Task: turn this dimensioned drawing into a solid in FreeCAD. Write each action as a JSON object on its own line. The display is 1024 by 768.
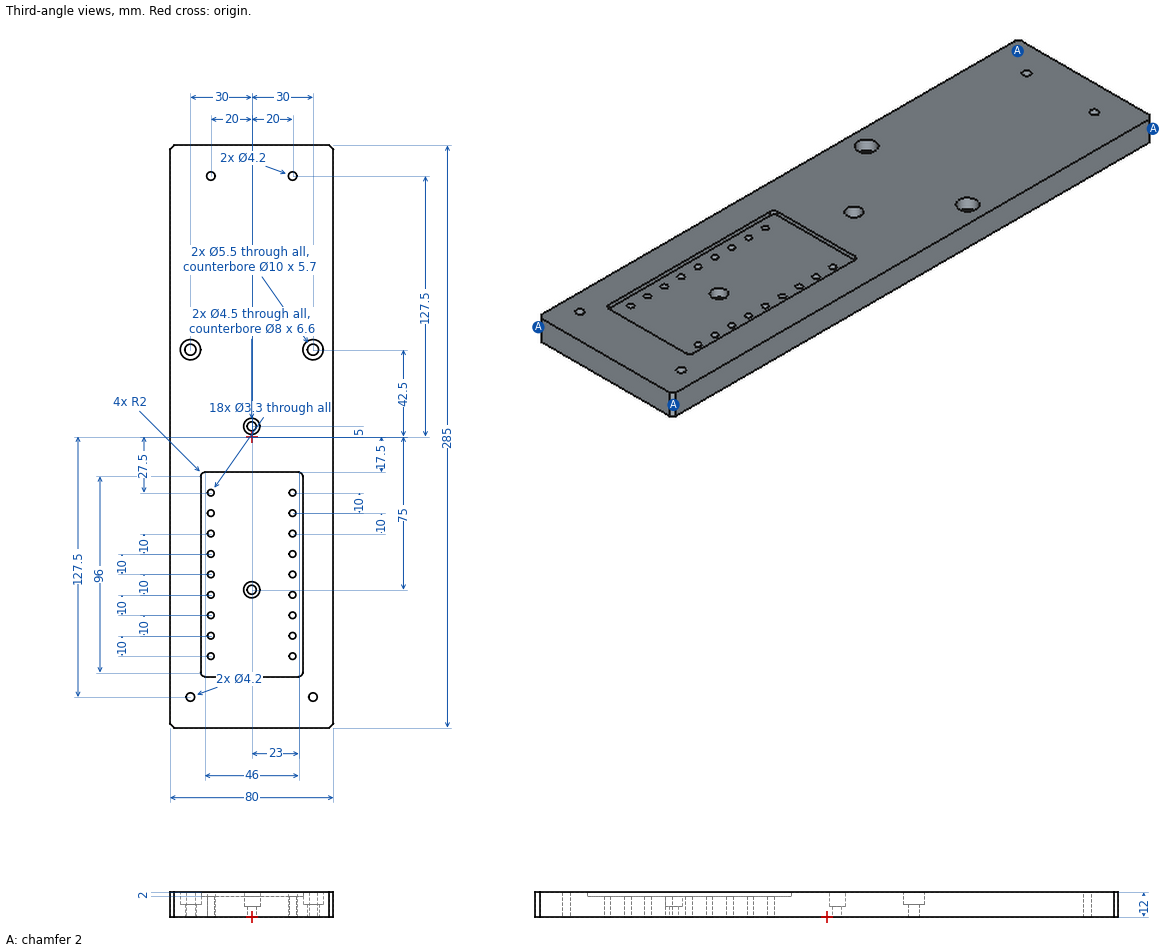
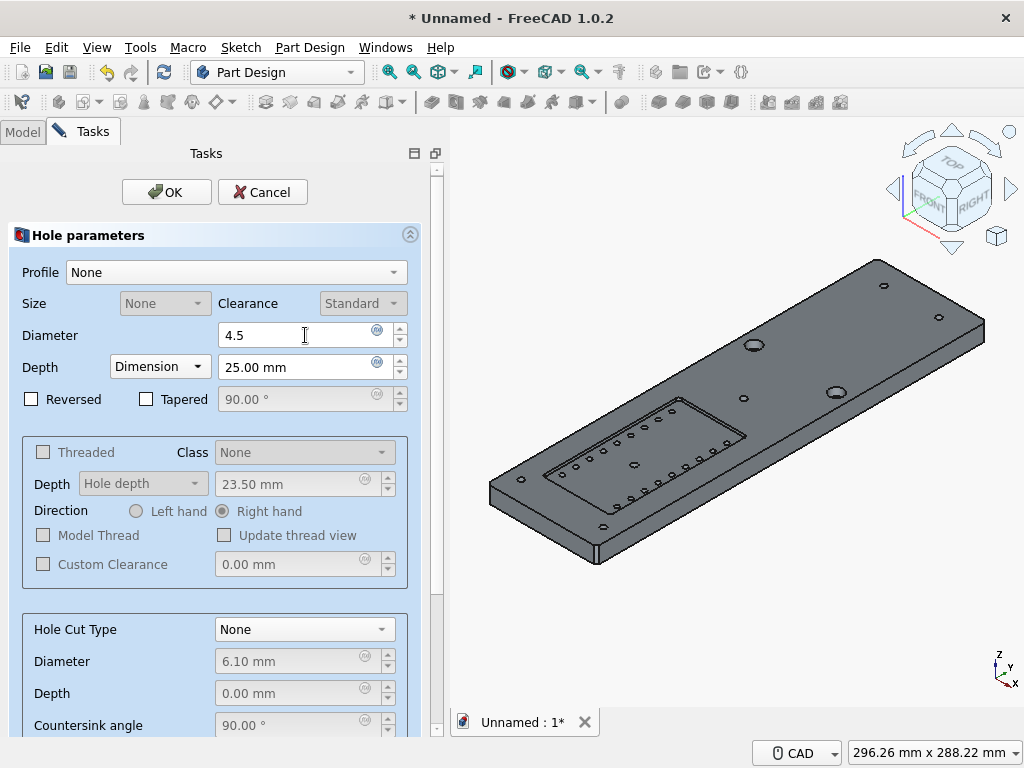
{"action": "left_click", "coordinate": [161, 366]}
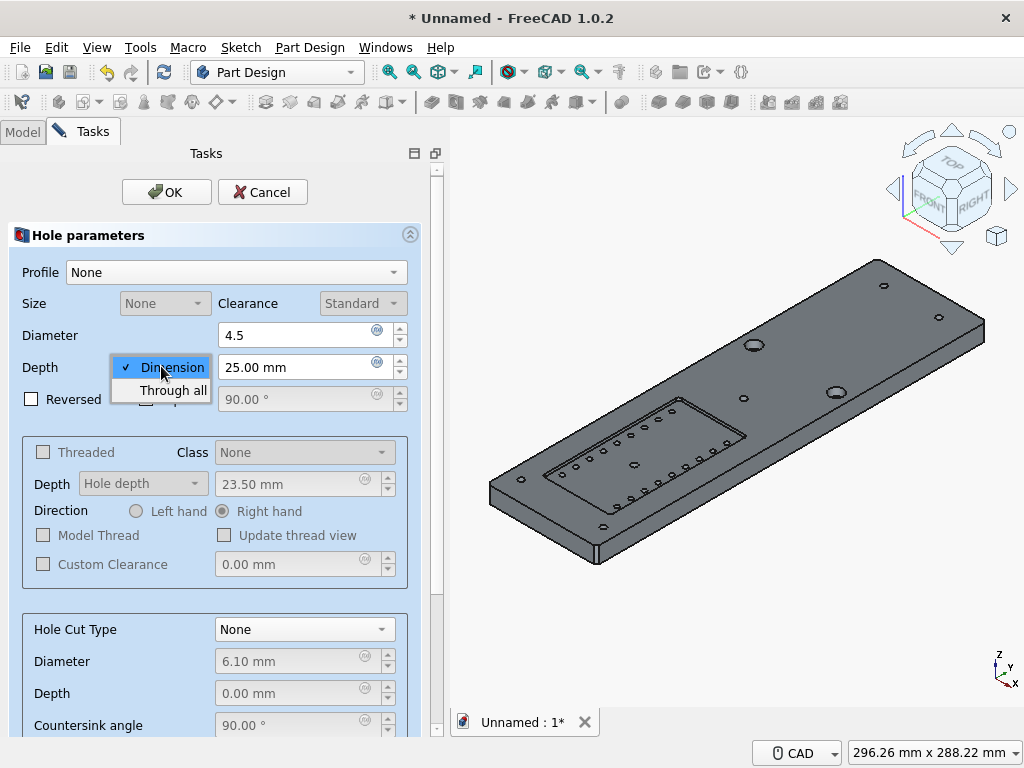
{"action": "left_click", "coordinate": [160, 390]}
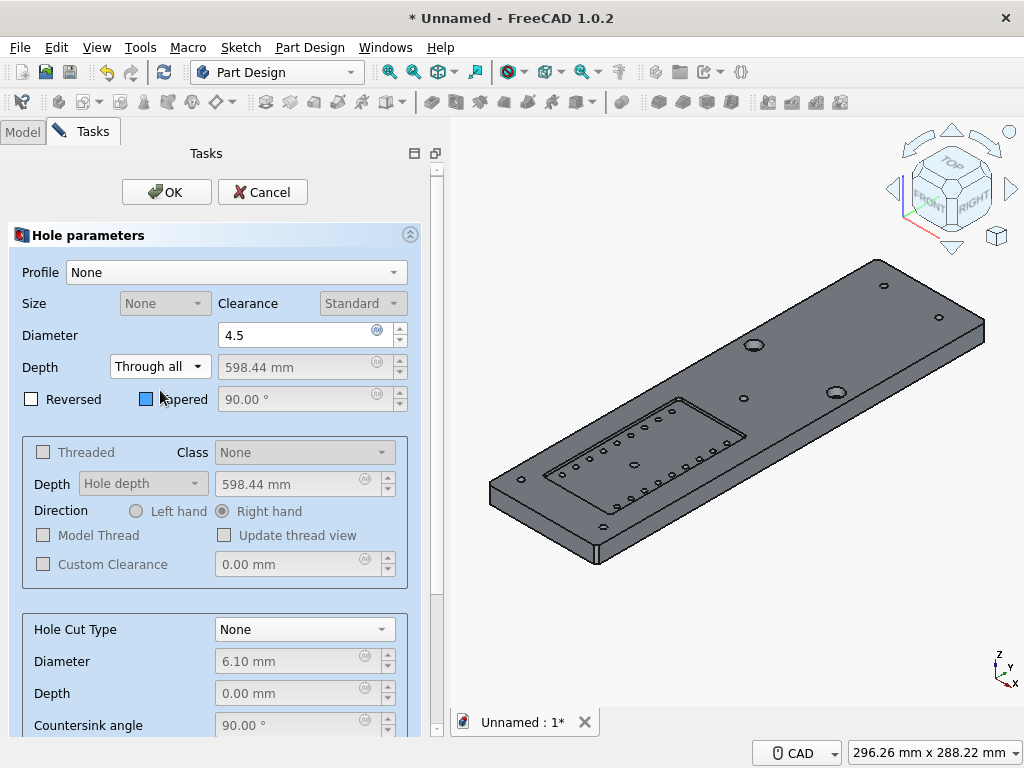
{"action": "left_click", "coordinate": [306, 630]}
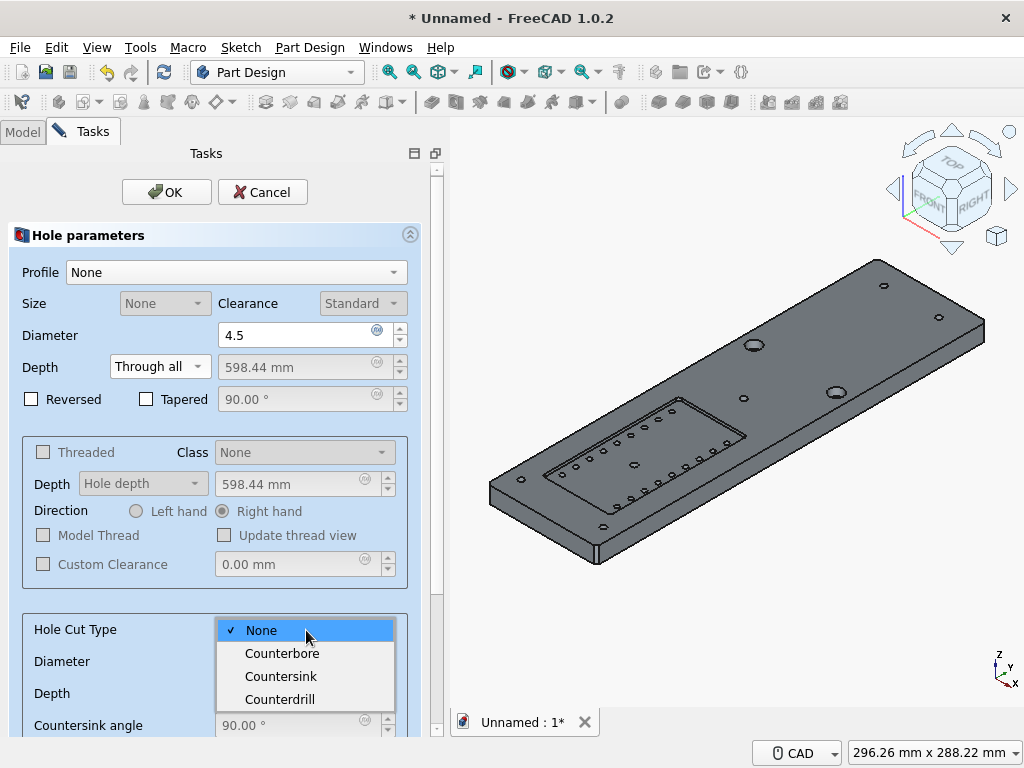
{"action": "left_click", "coordinate": [304, 654]}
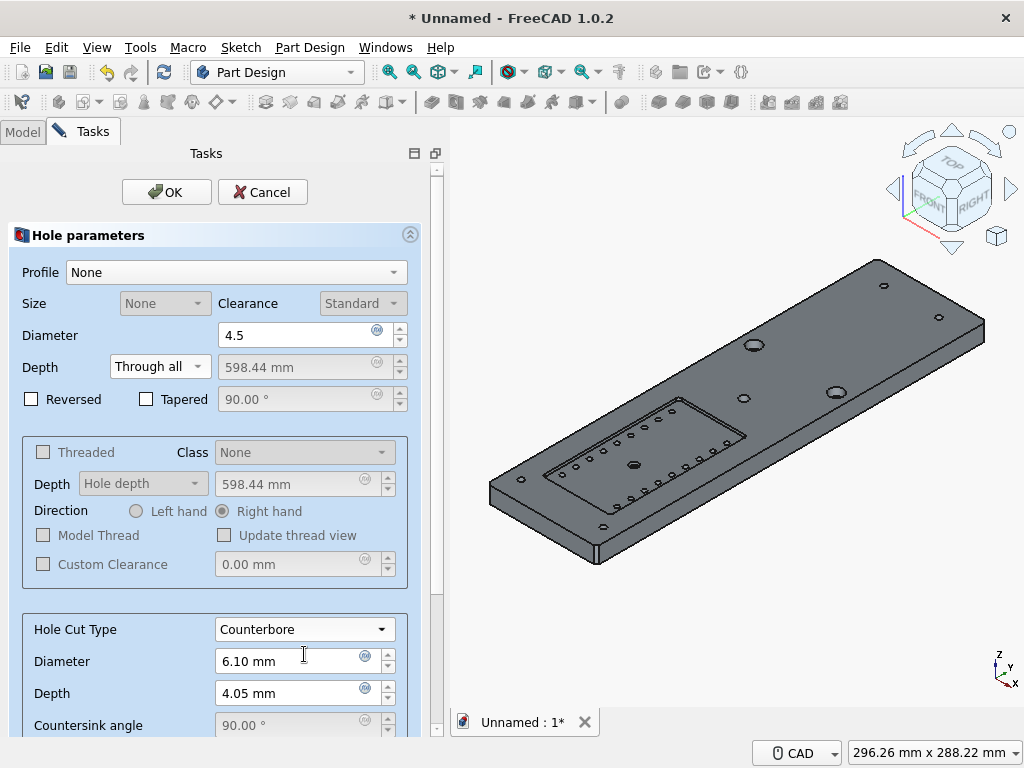
{"action": "triple_click", "coordinate": [298, 661]}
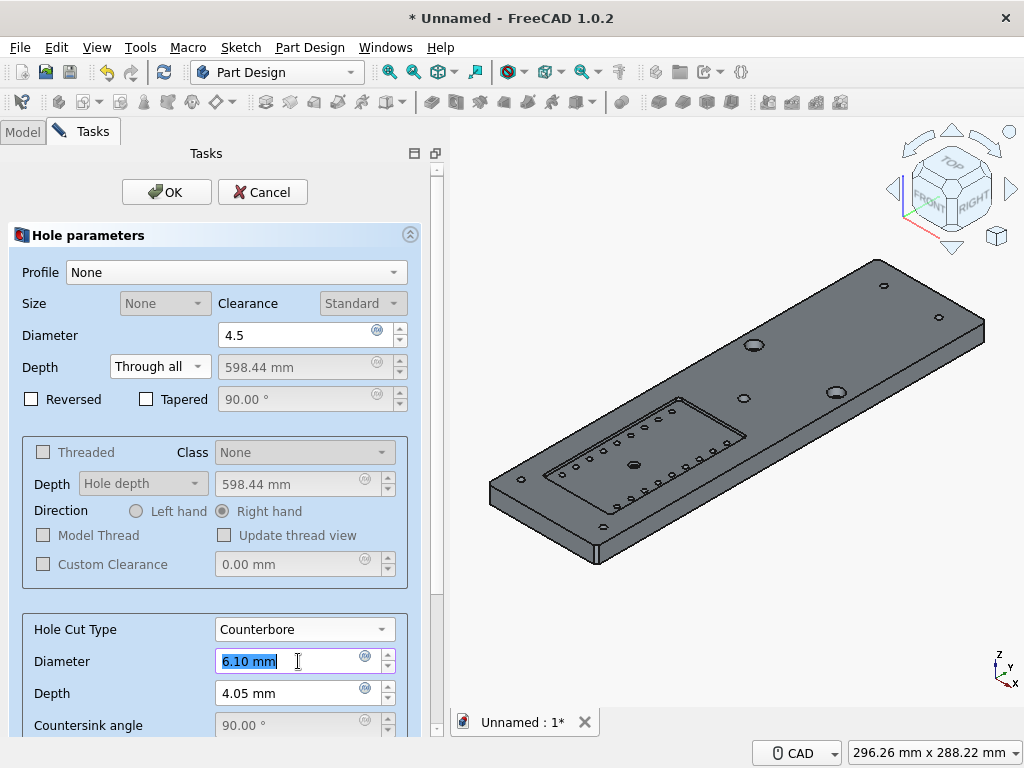
{"action": "type", "text": "8"}
{"action": "key", "text": "Tab"}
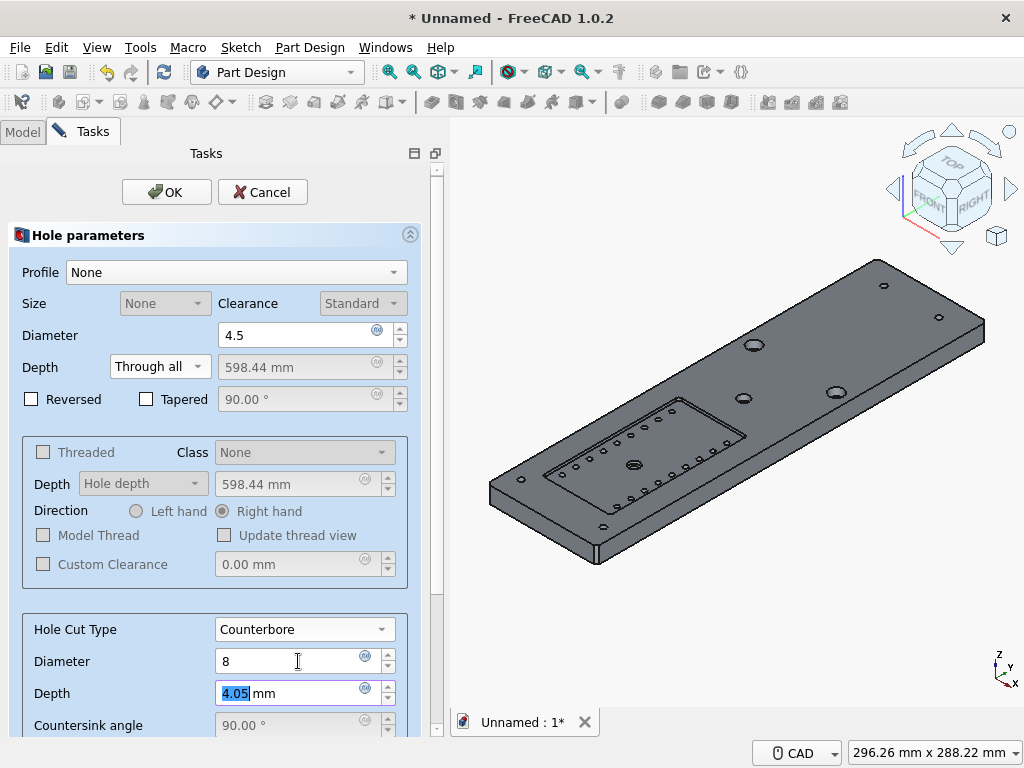
{"action": "type", "text": "6.6"}
{"action": "key", "text": "Tab"}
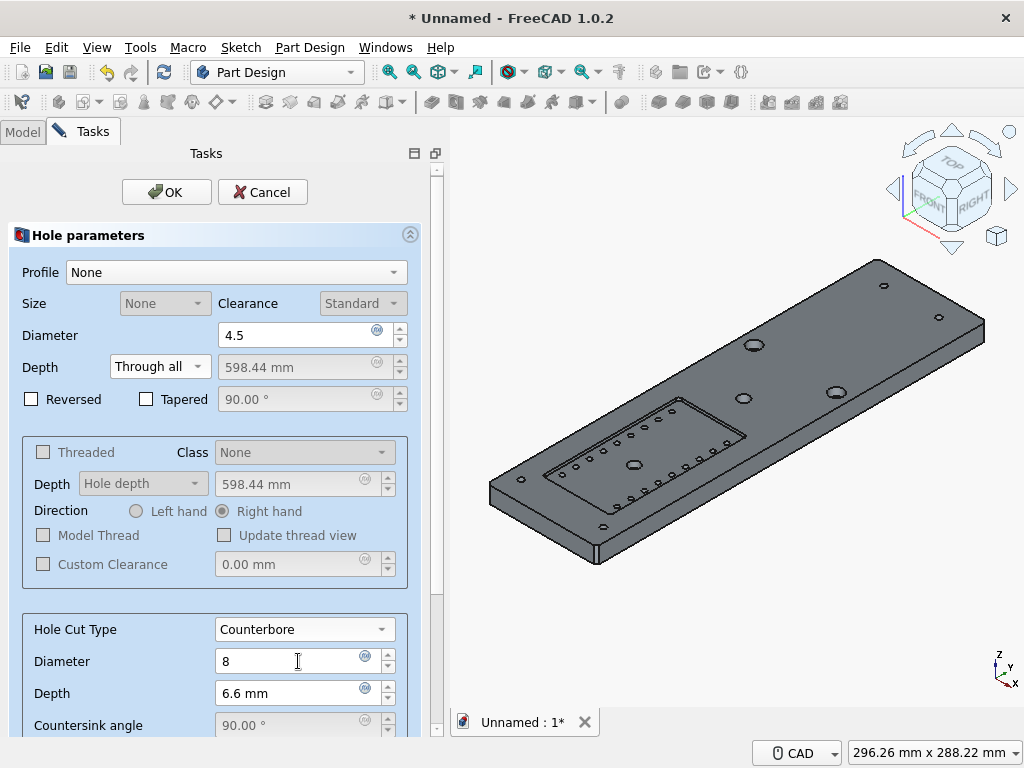
{"action": "left_click", "coordinate": [167, 192]}